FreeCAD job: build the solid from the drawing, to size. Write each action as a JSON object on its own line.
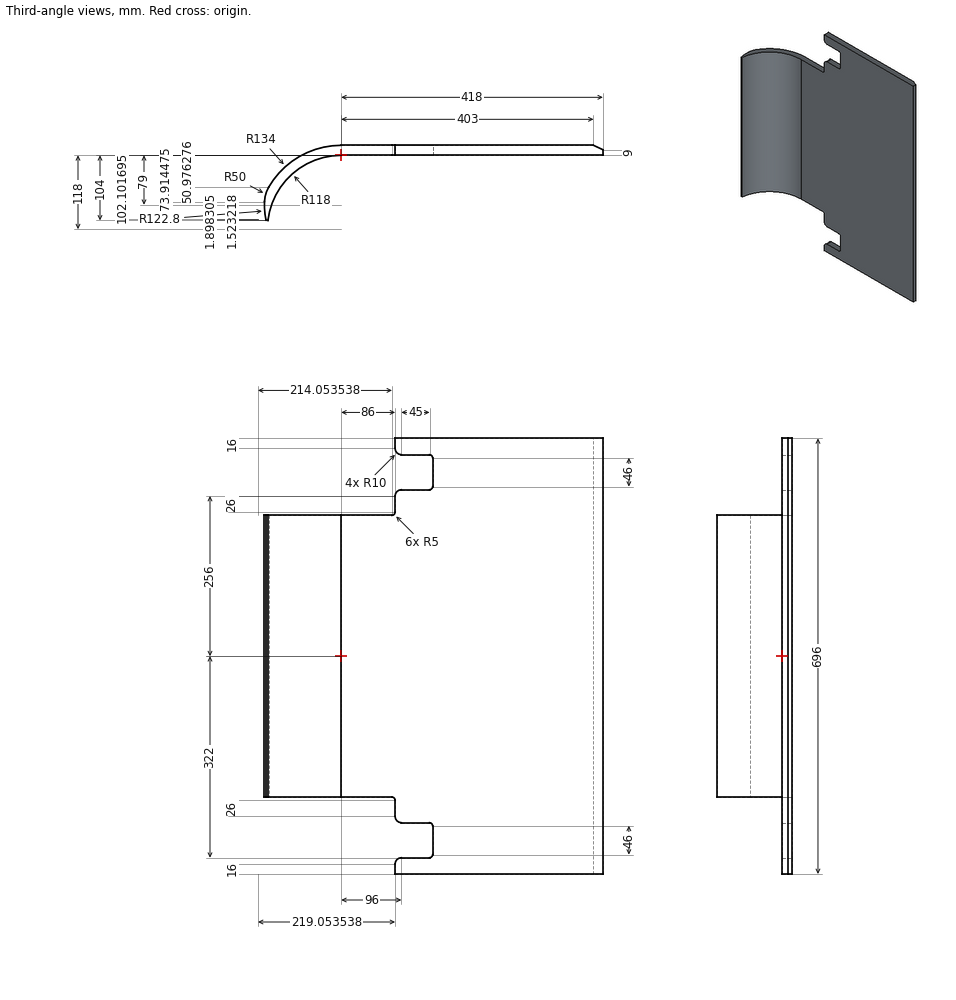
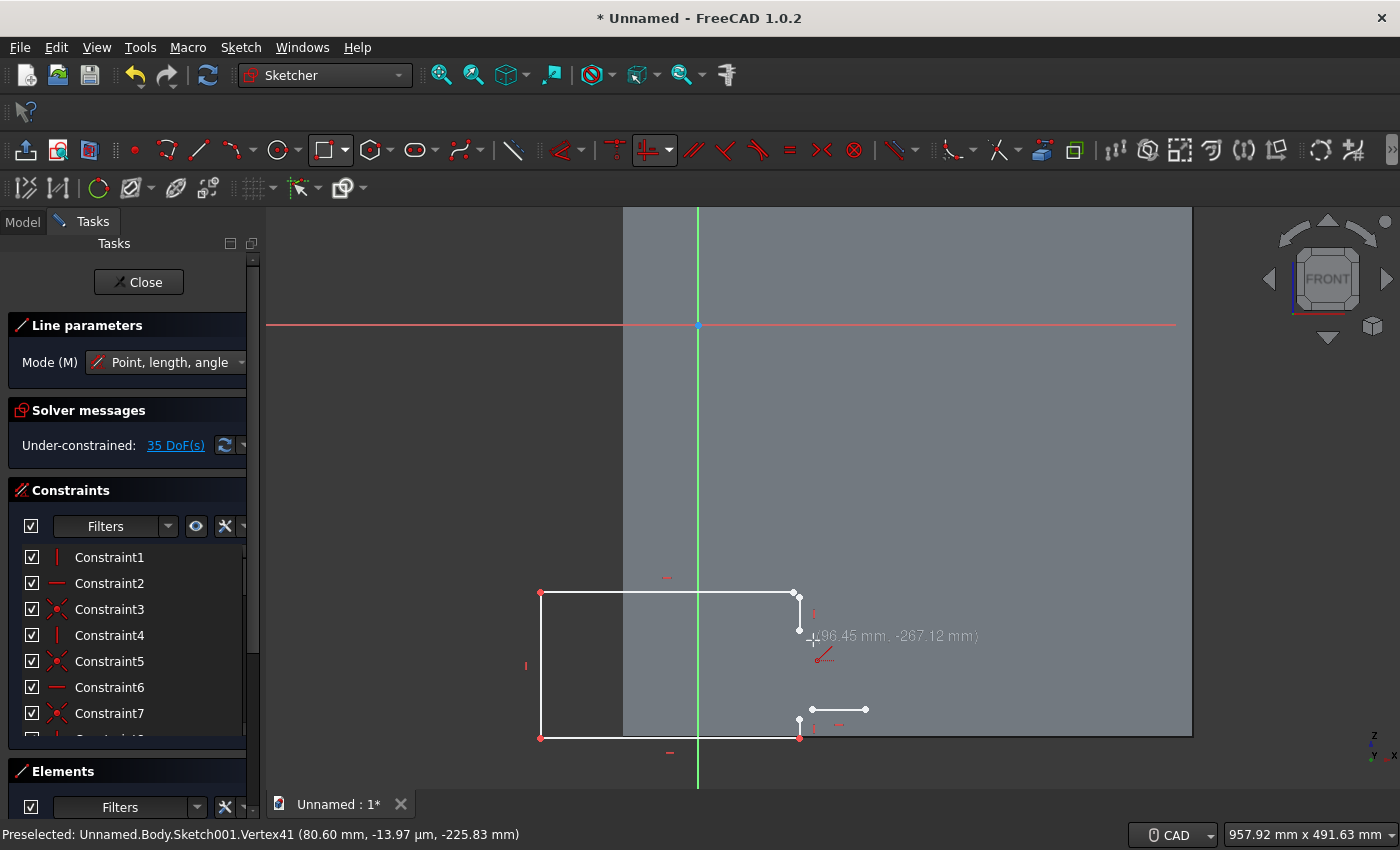
{"action": "left_click", "coordinate": [812, 640]}
{"action": "left_click", "coordinate": [865, 640]}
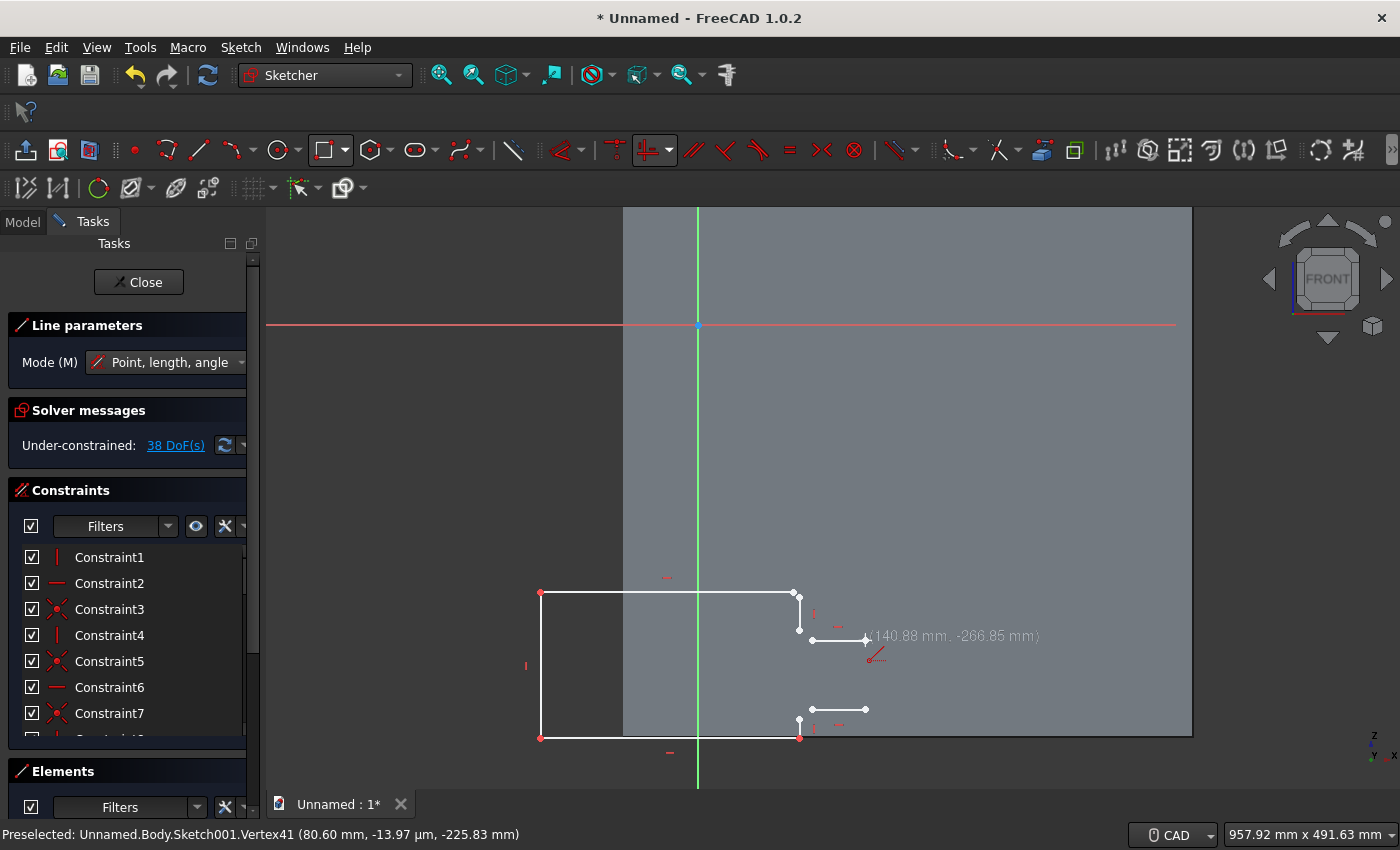
{"action": "scroll", "coordinate": [871, 646], "scroll_direction": "up", "scroll_amount": 4}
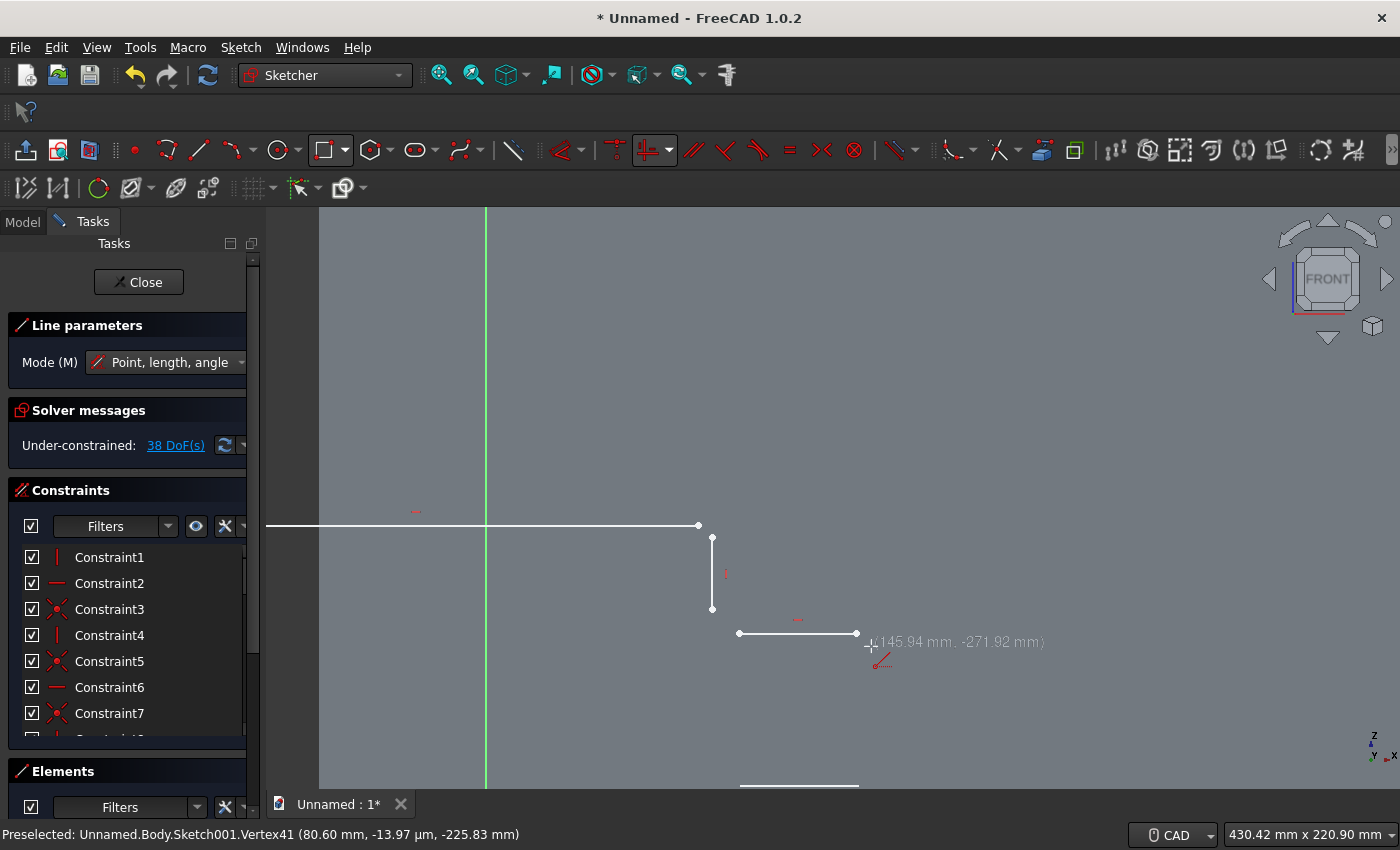
{"action": "left_click", "coordinate": [870, 645]}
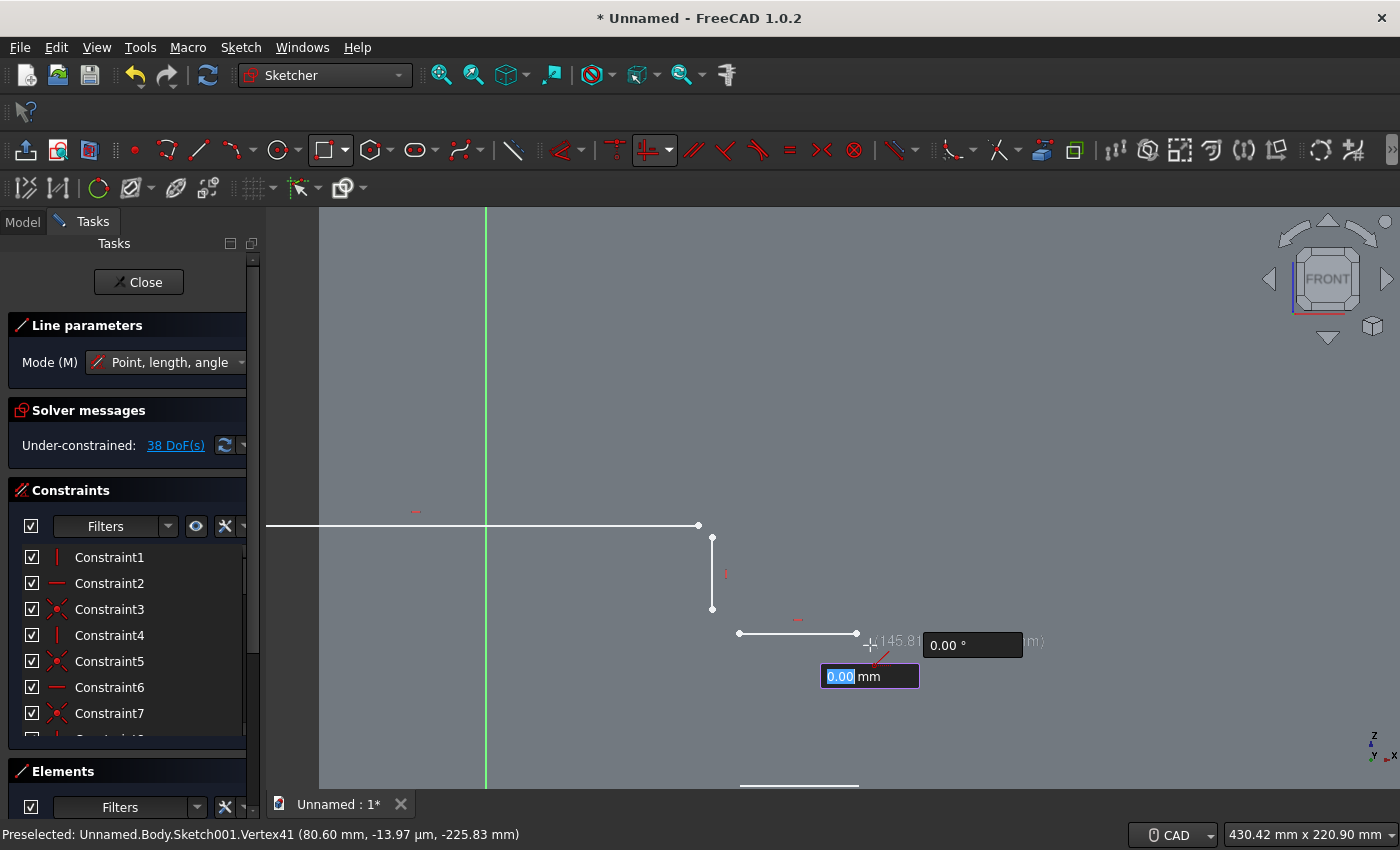
{"action": "scroll", "coordinate": [831, 641], "scroll_direction": "down", "scroll_amount": 8}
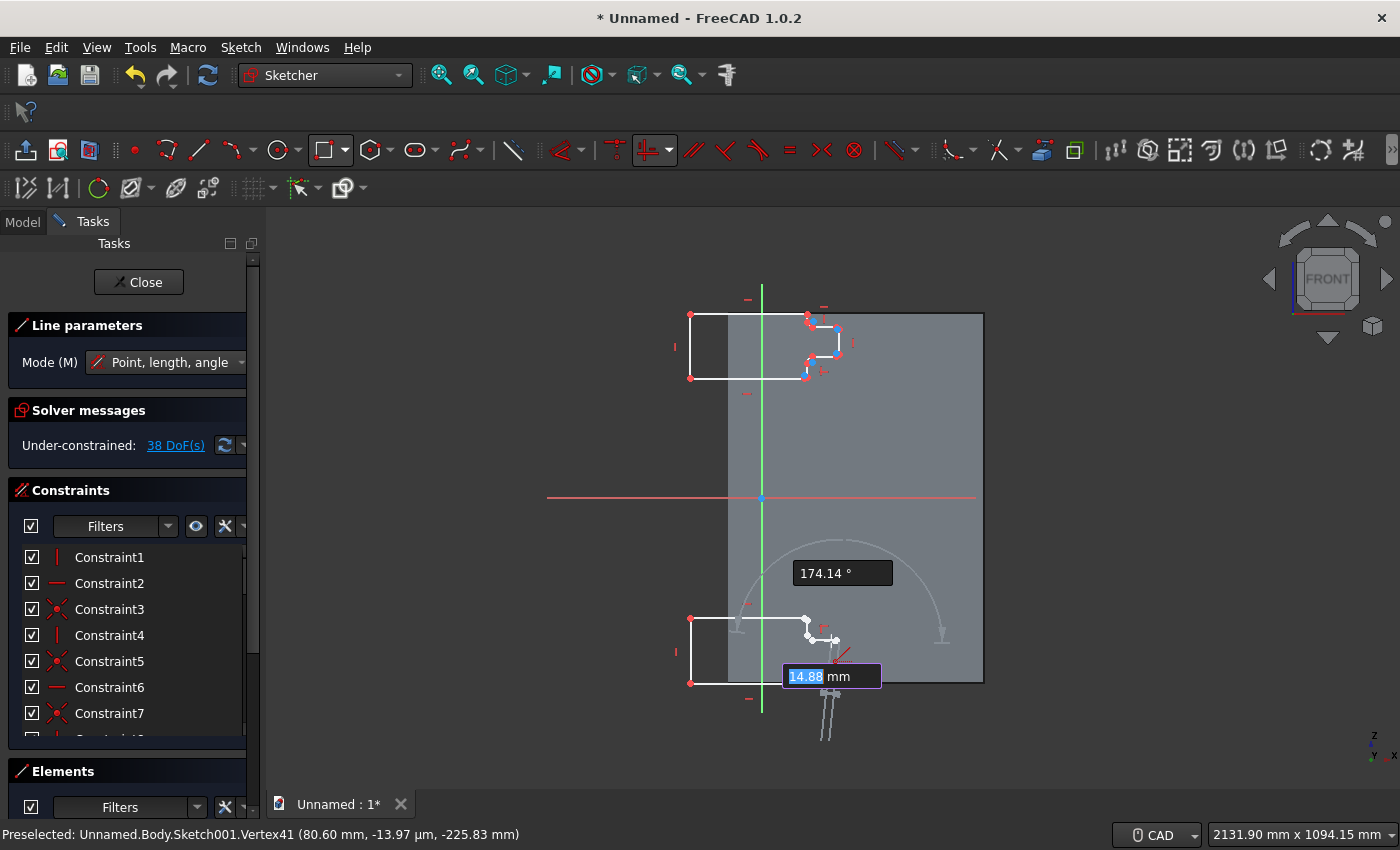
{"action": "scroll", "coordinate": [839, 667], "scroll_direction": "up", "scroll_amount": 8}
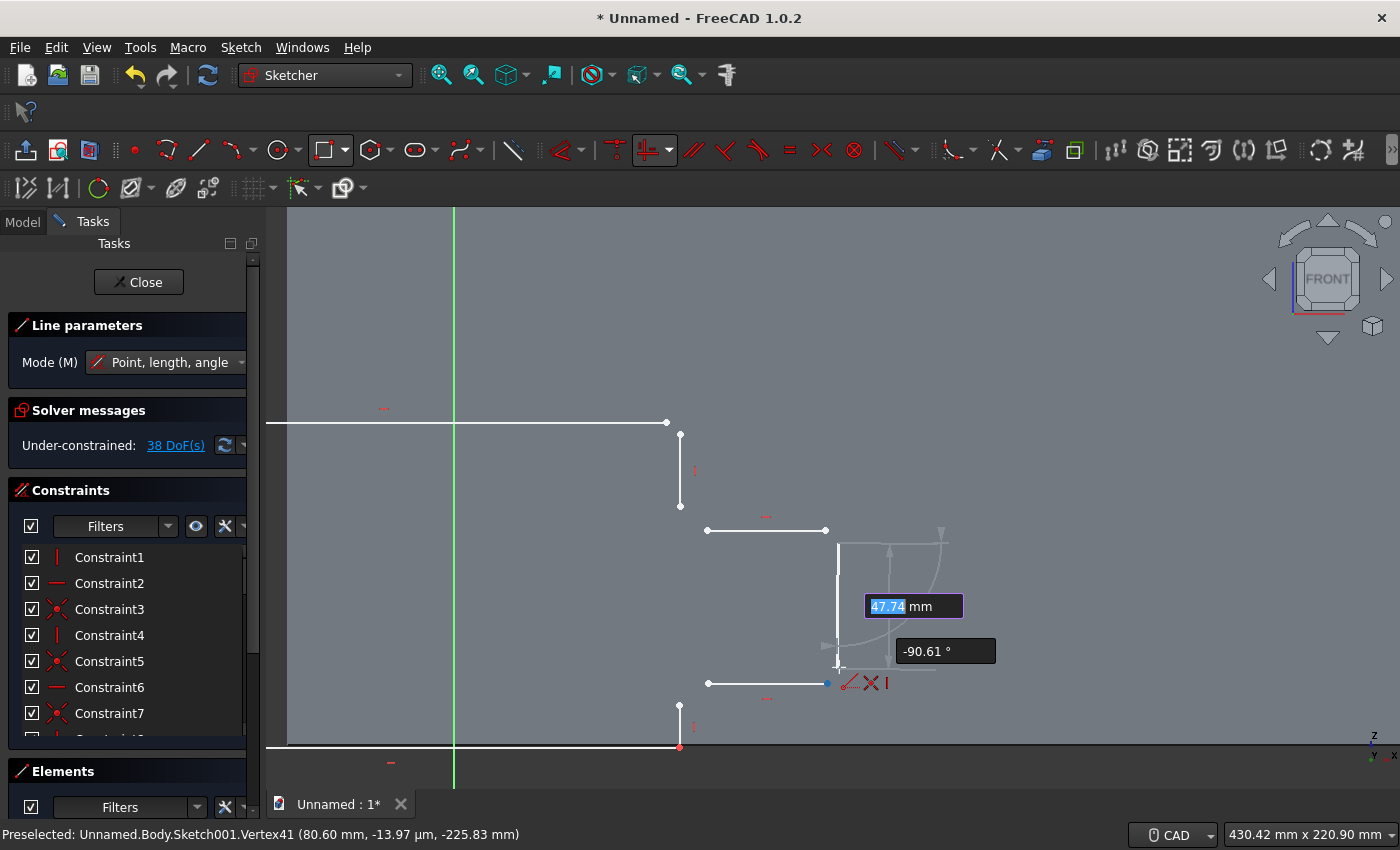
{"action": "left_click", "coordinate": [838, 663]}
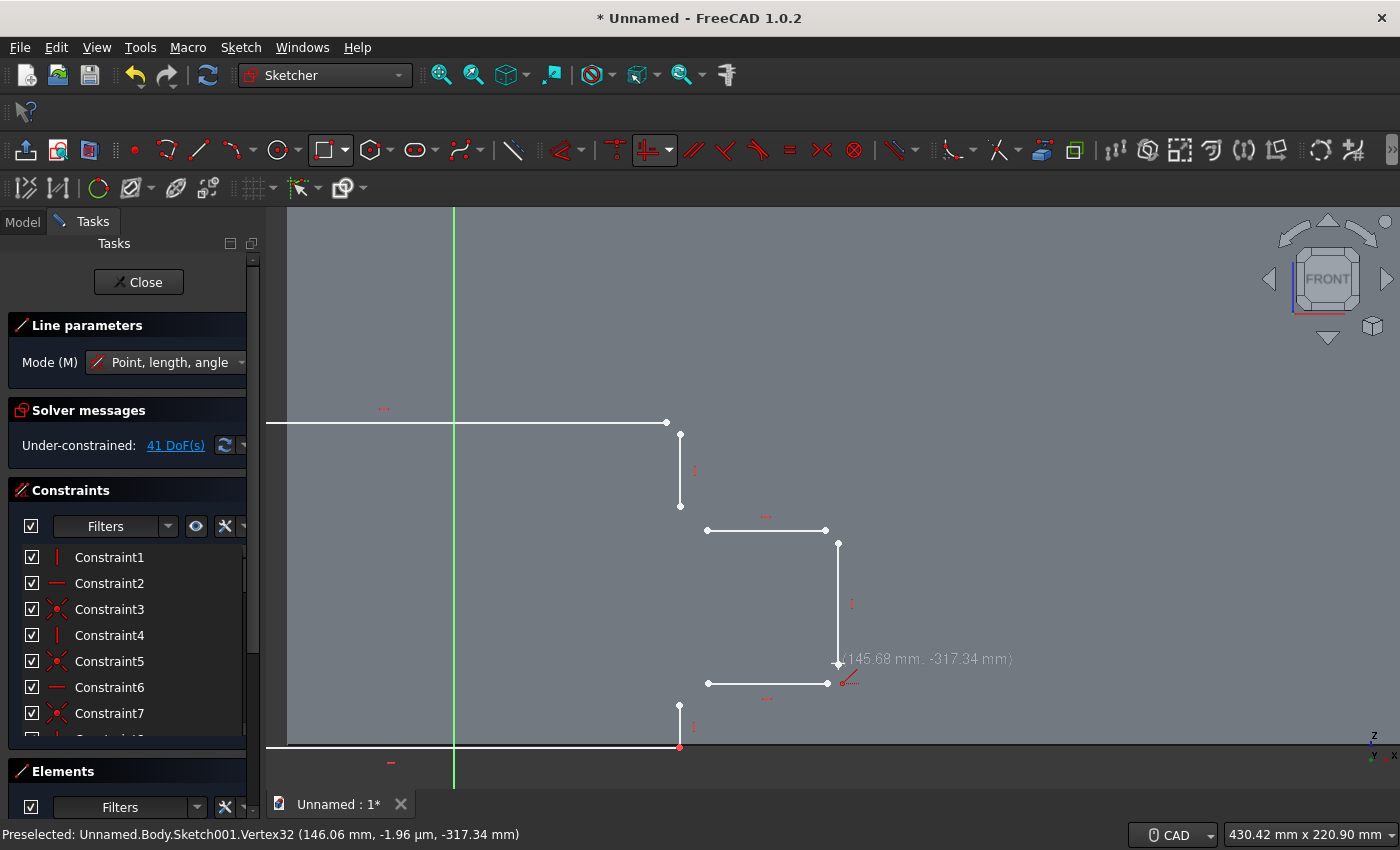
{"action": "left_click", "coordinate": [232, 150]}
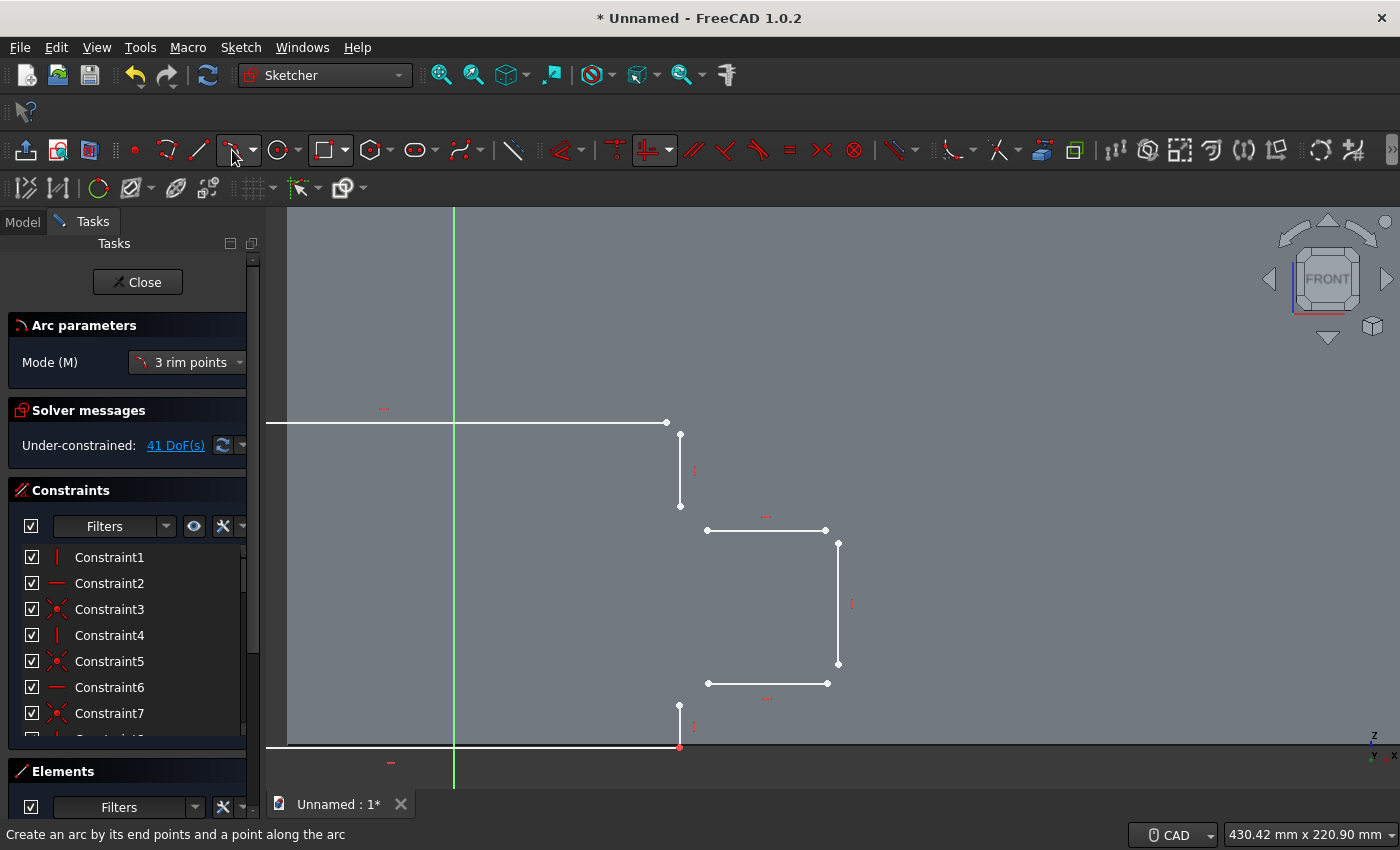
{"action": "left_click", "coordinate": [708, 684]}
{"action": "left_click", "coordinate": [680, 706]}